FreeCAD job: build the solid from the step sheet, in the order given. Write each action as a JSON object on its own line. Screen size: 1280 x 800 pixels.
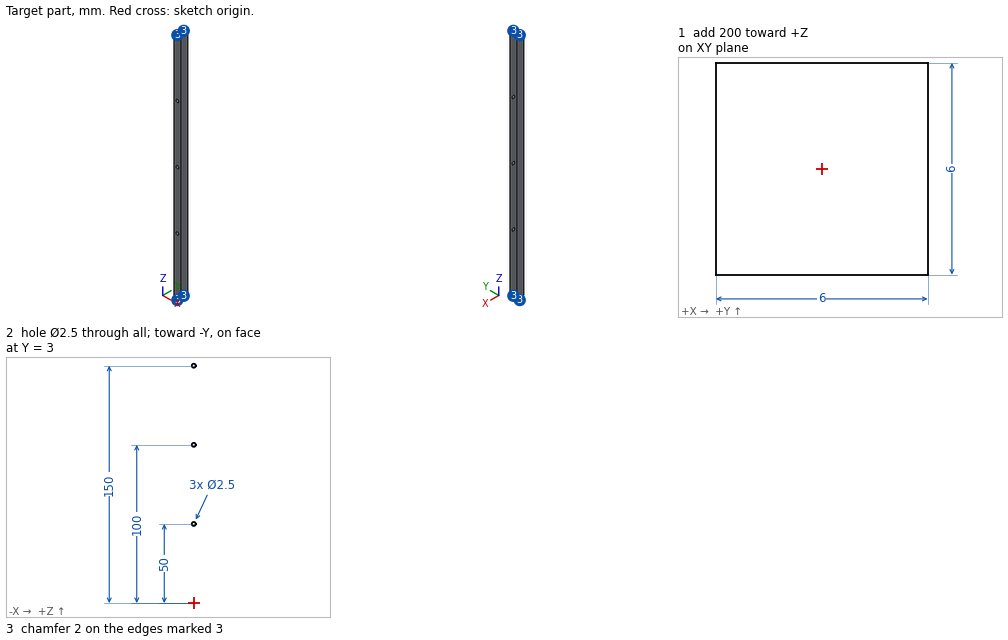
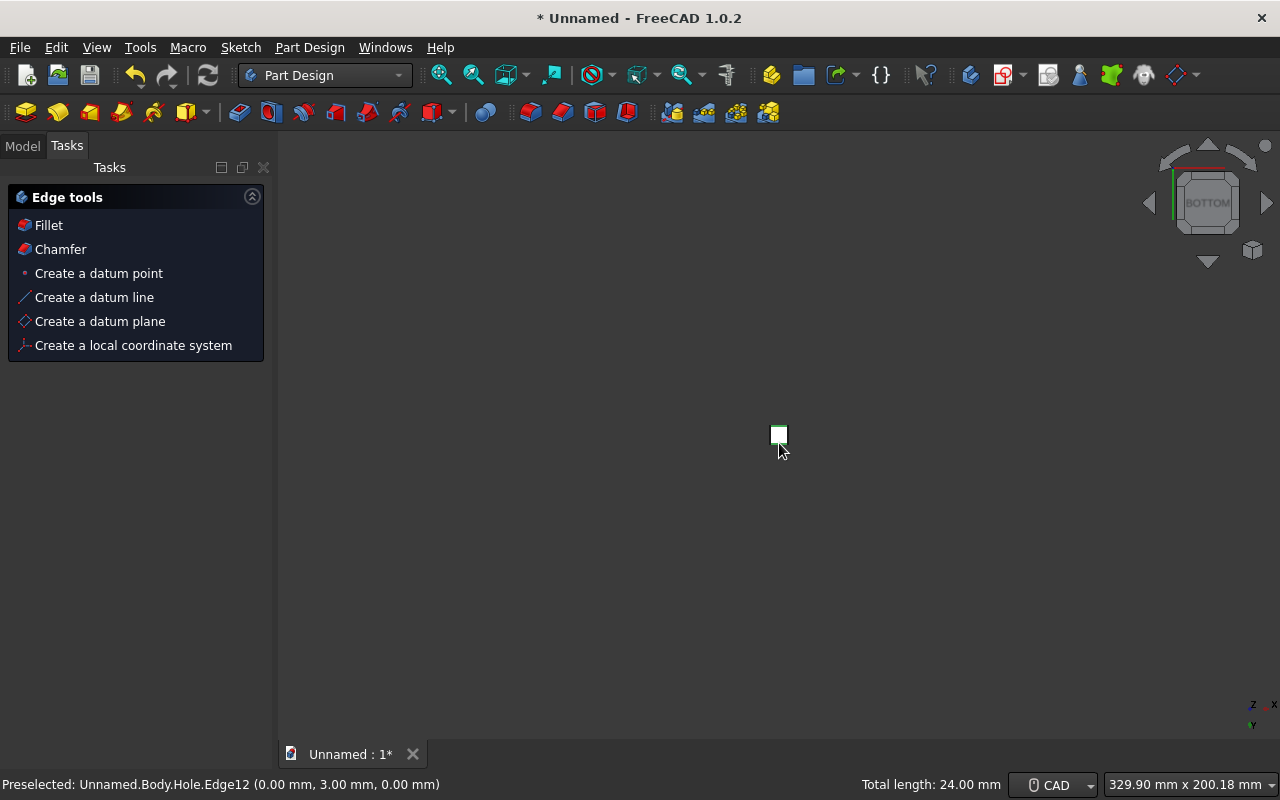
{"action": "left_click", "coordinate": [564, 112]}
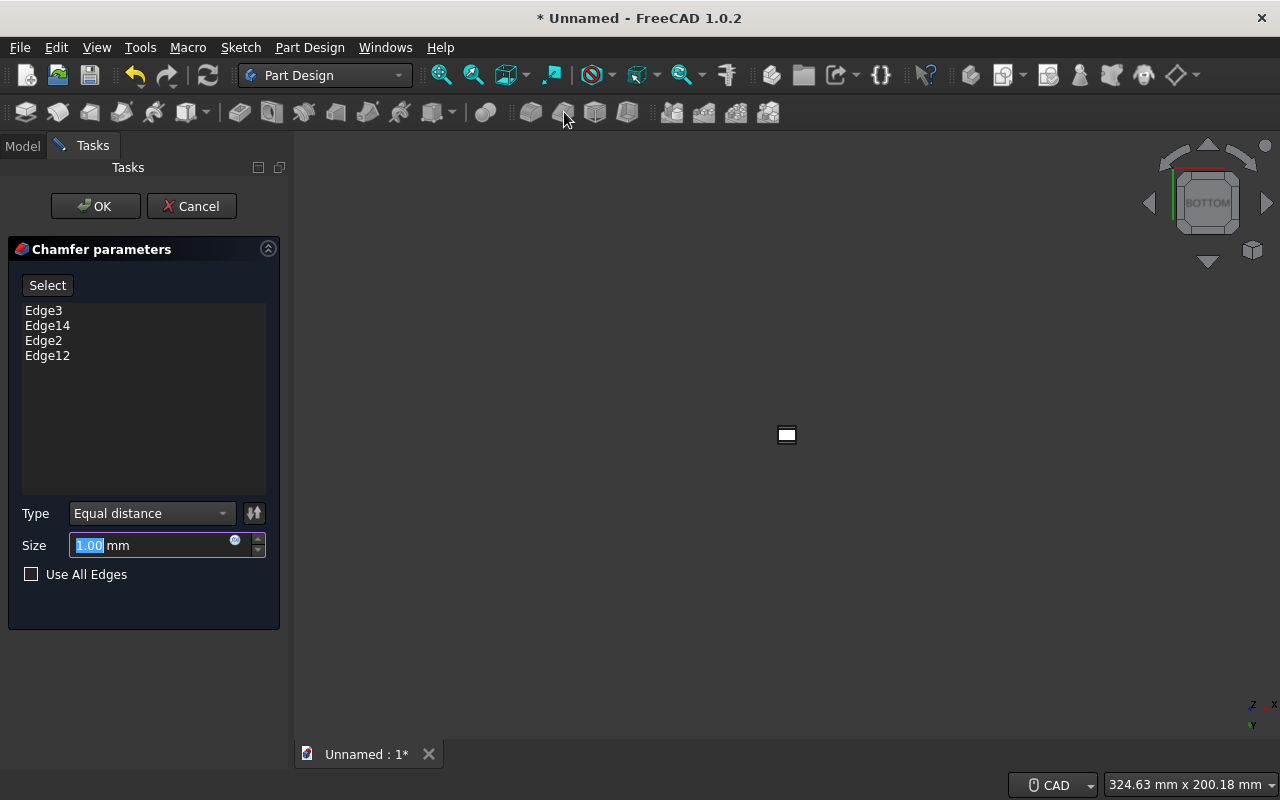
{"action": "type", "text": "2"}
{"action": "key", "text": "Tab"}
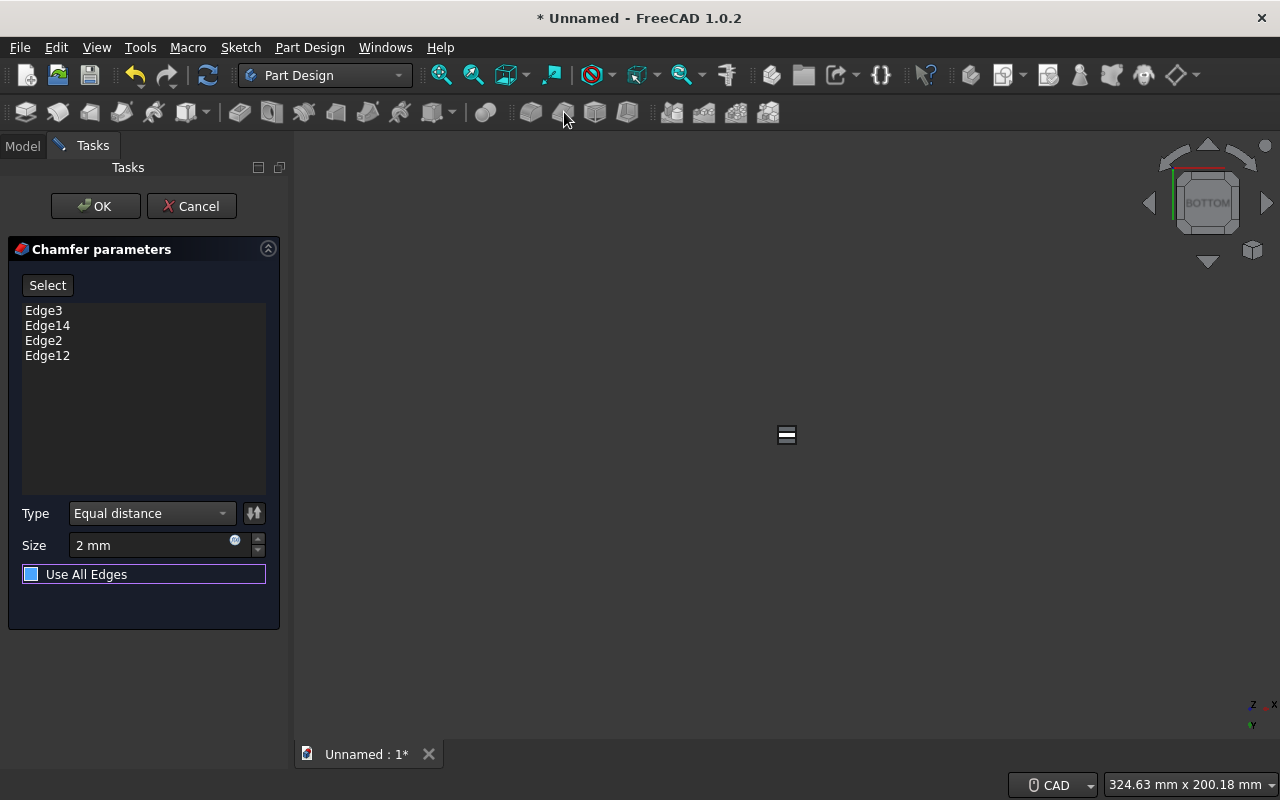
{"action": "left_click", "coordinate": [96, 206]}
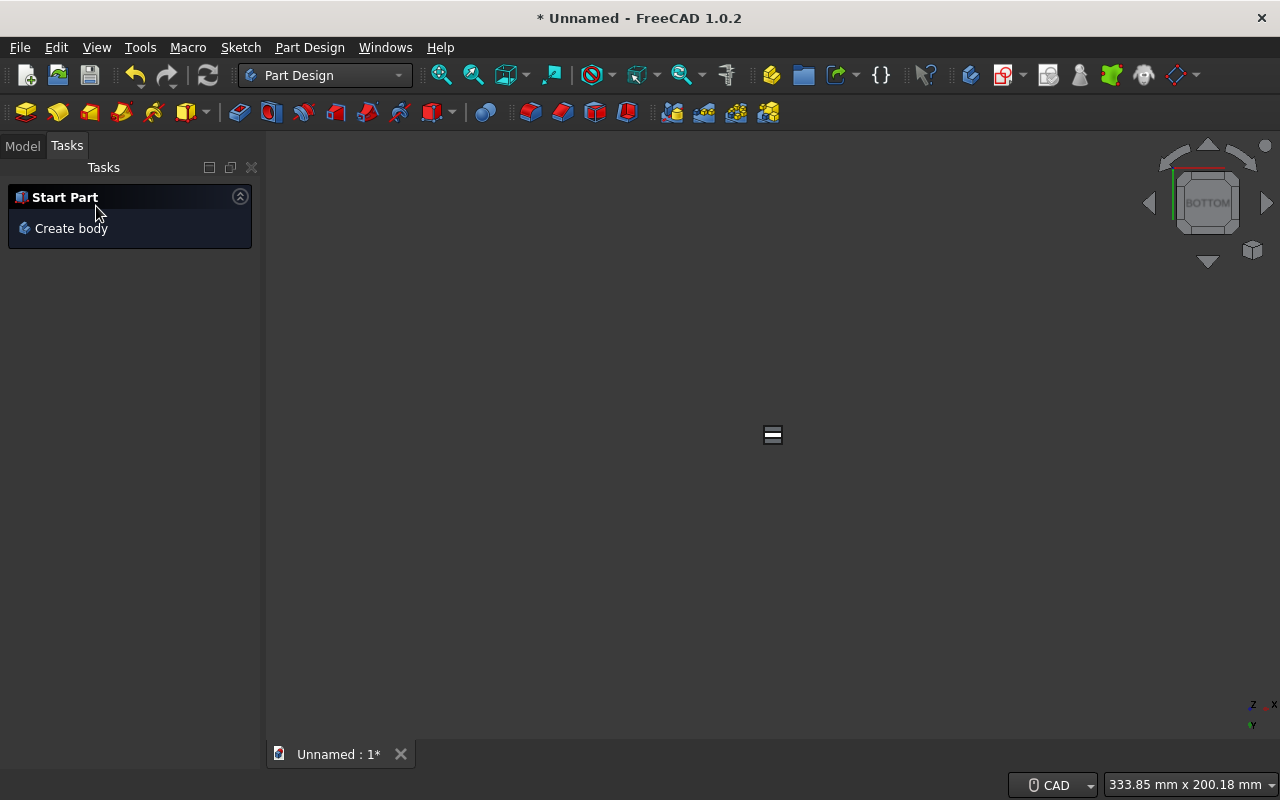
{"action": "key", "text": "0"}